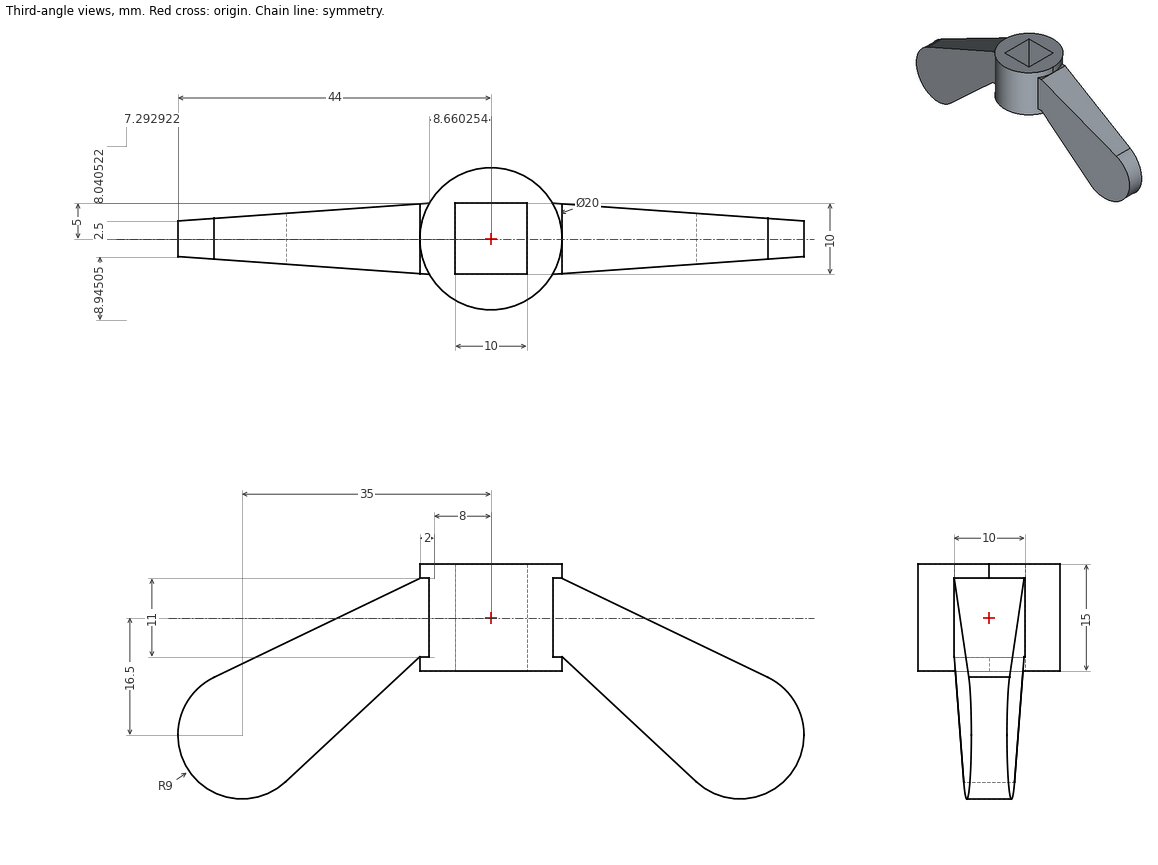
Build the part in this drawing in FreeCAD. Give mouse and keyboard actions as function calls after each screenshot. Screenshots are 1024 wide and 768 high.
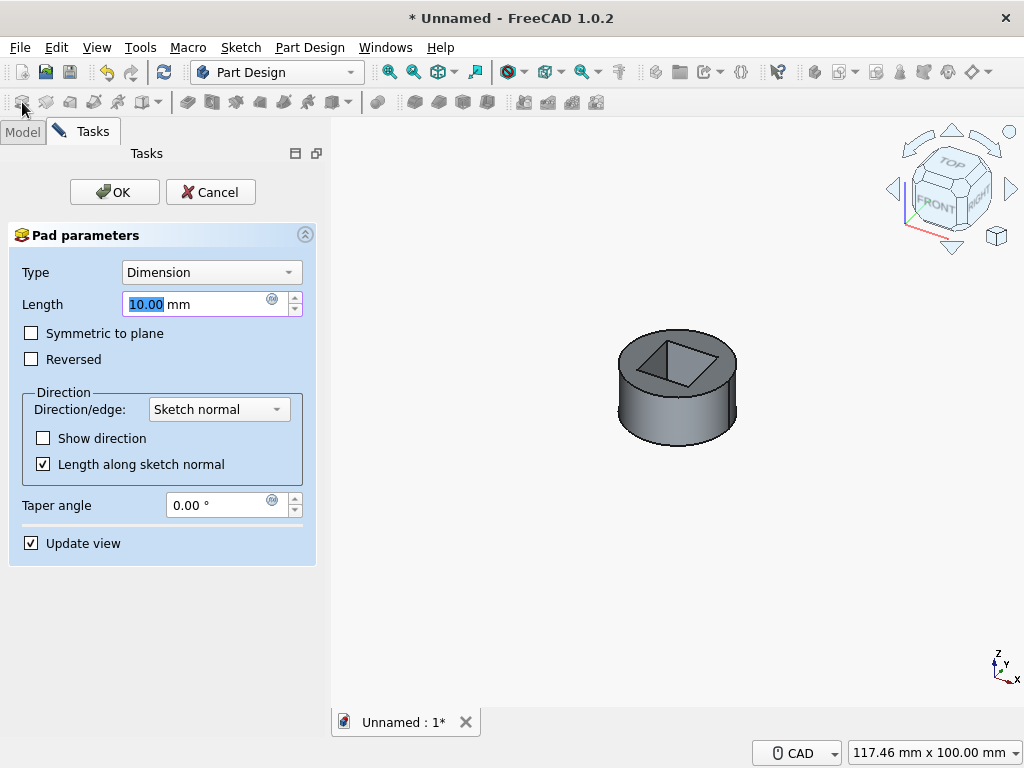
text(15)
key(Tab)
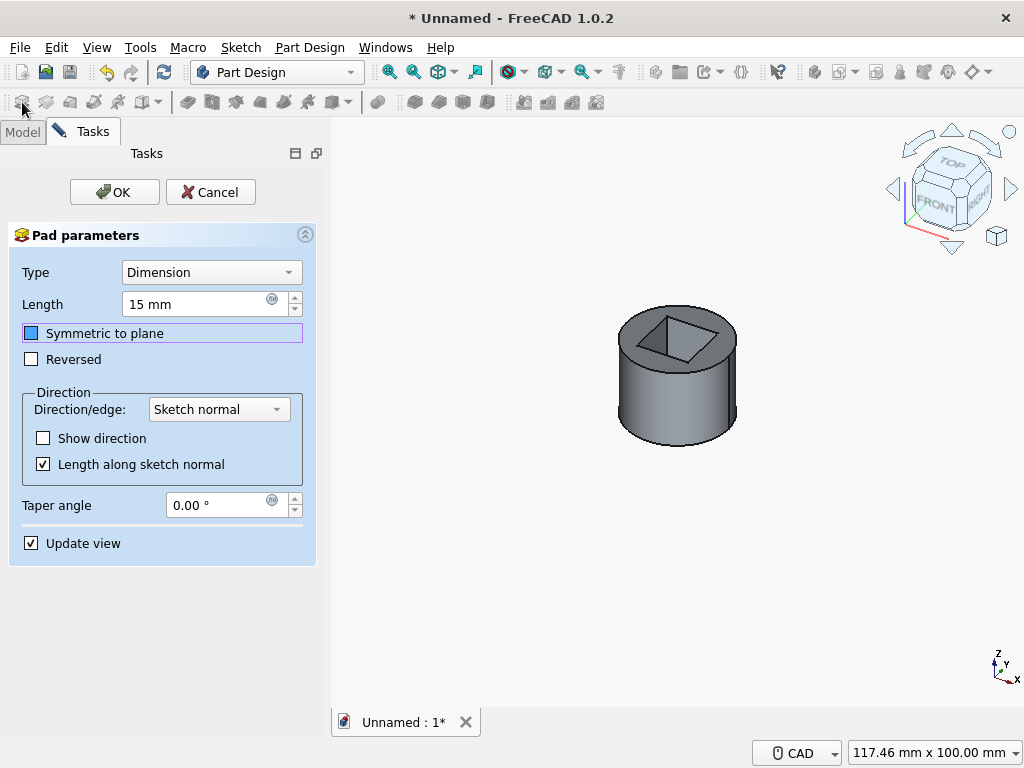
click(30, 333)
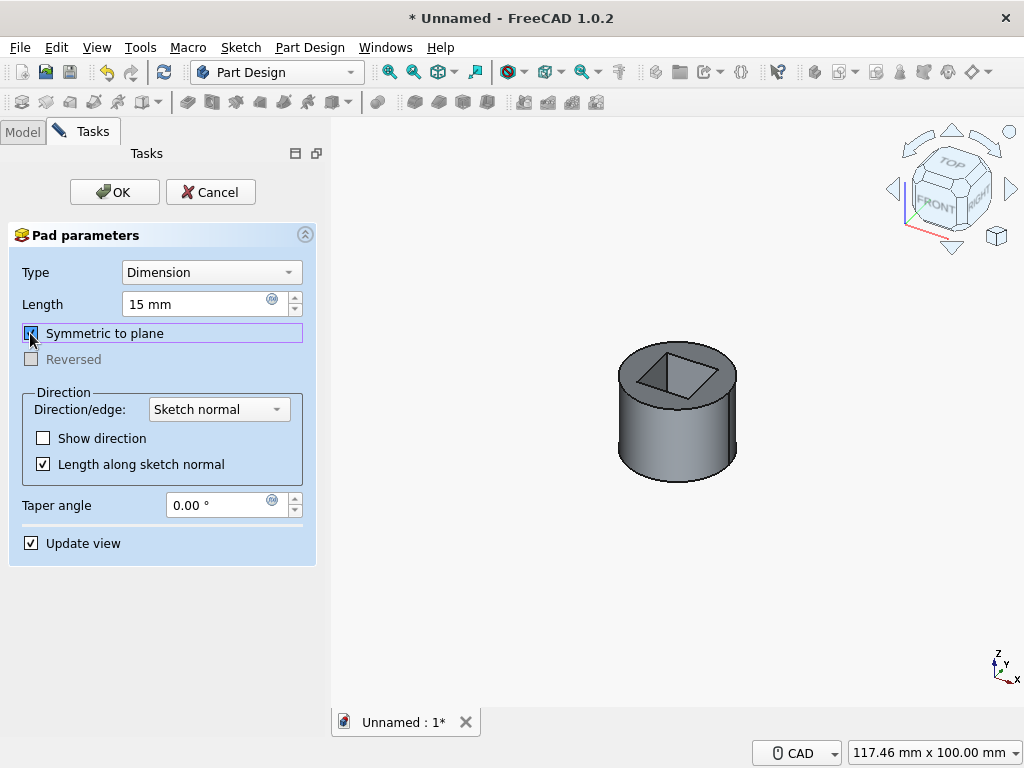
click(115, 192)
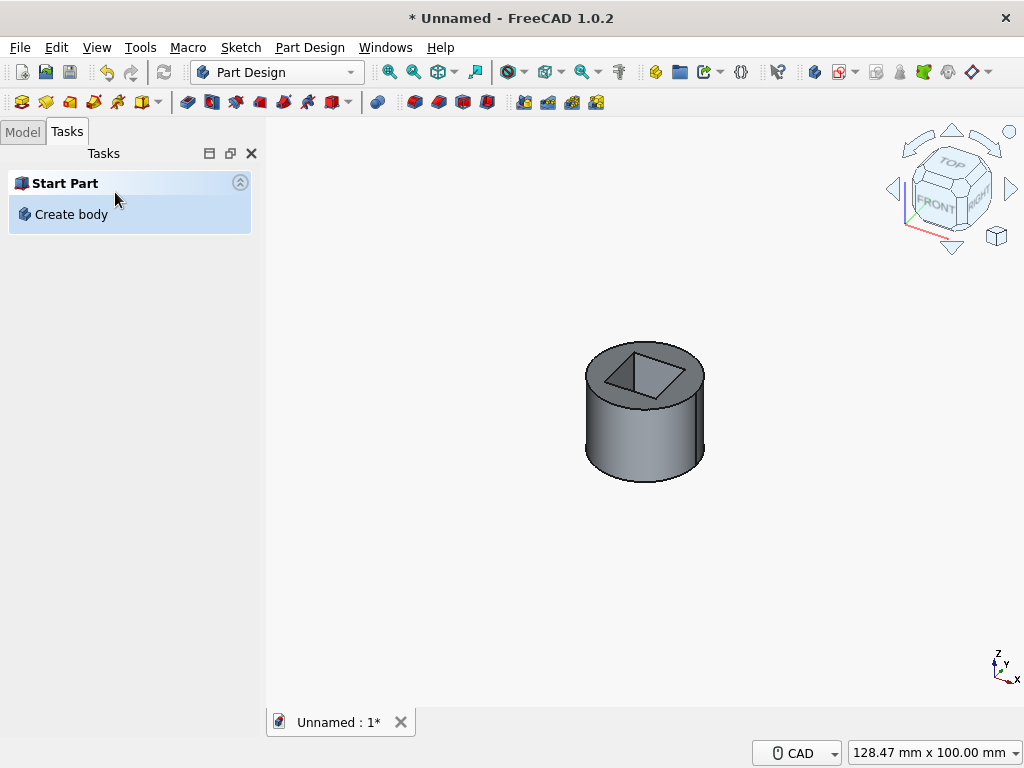
click(390, 72)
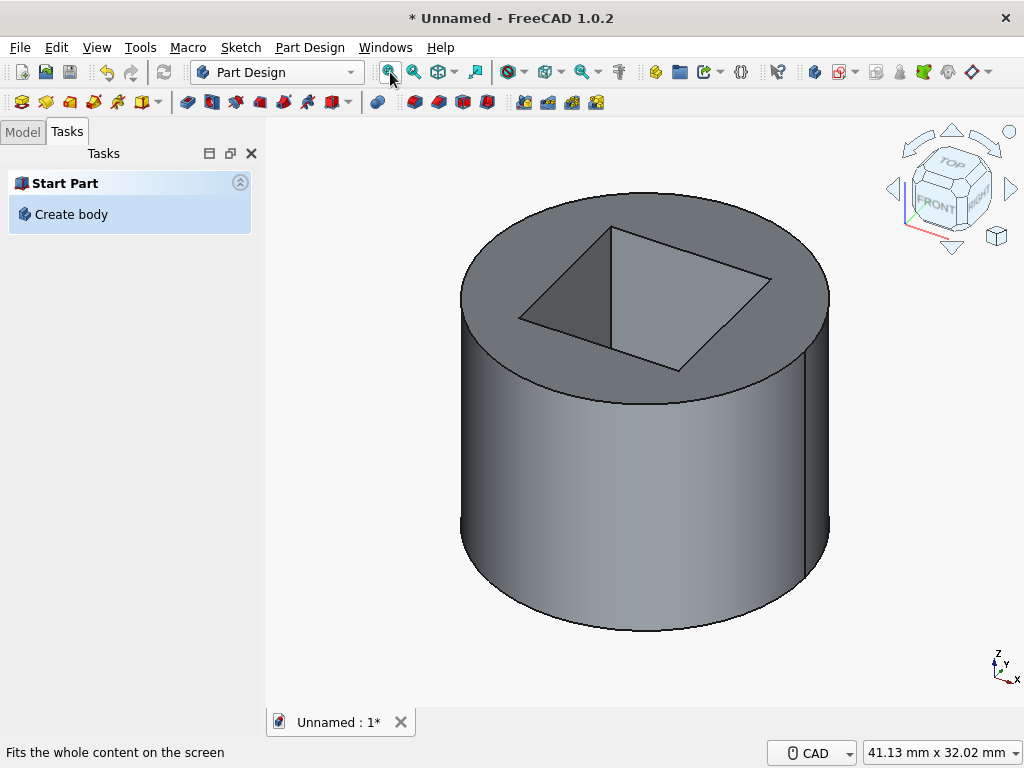
click(840, 72)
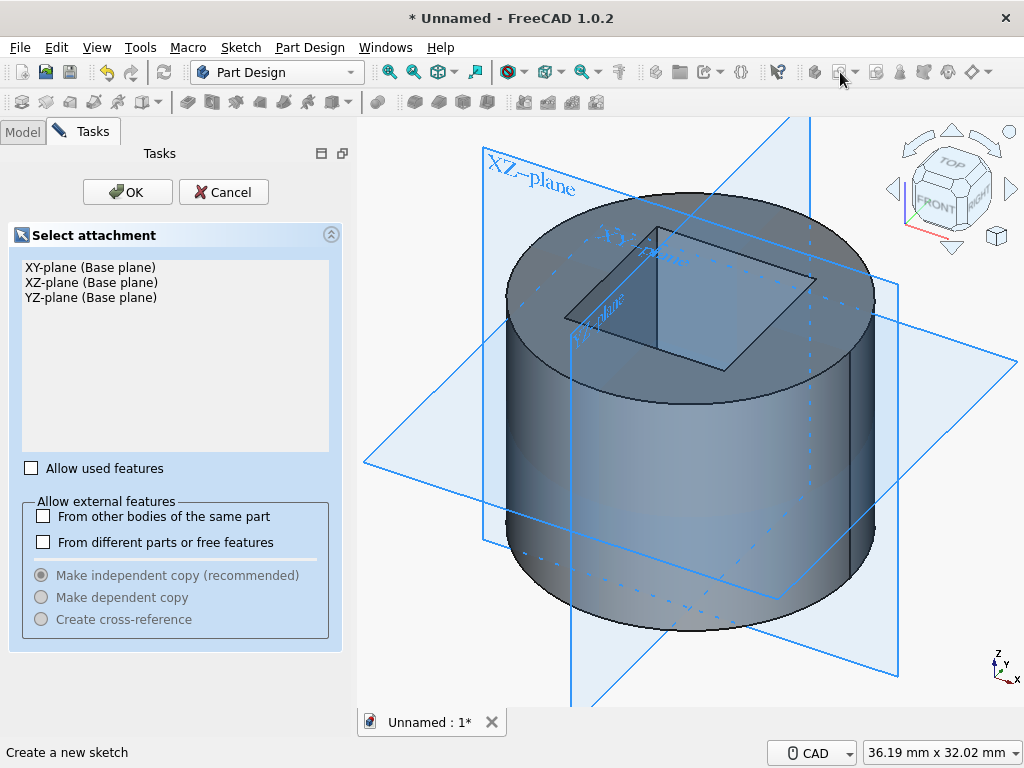
click(82, 282)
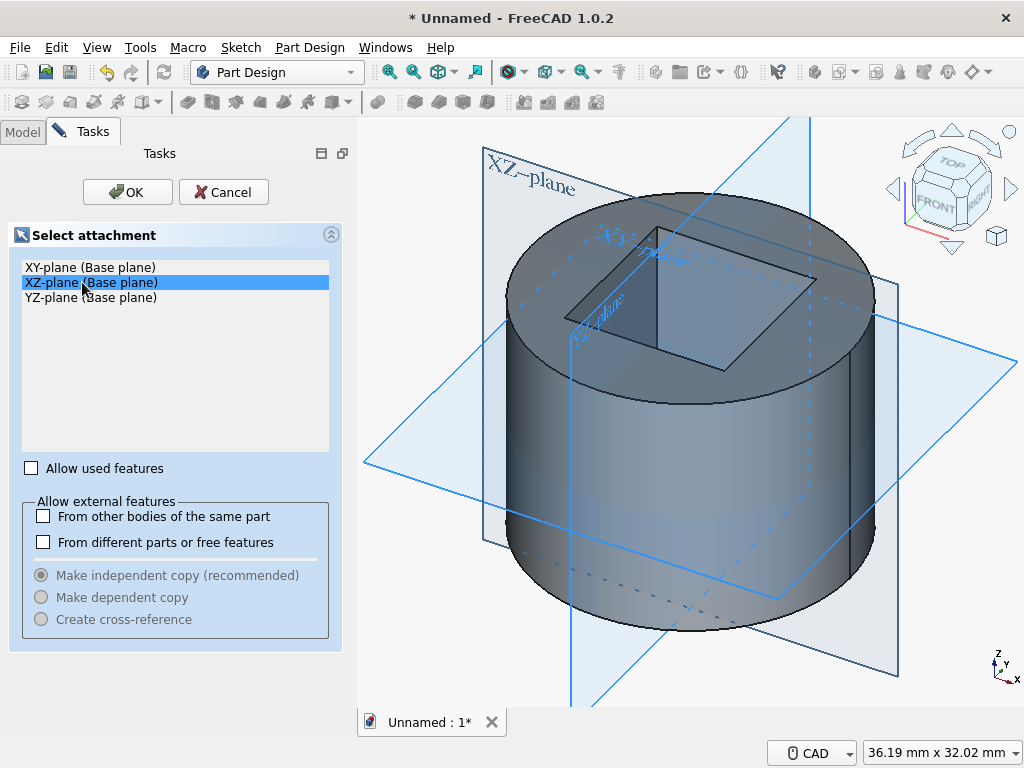
click(128, 192)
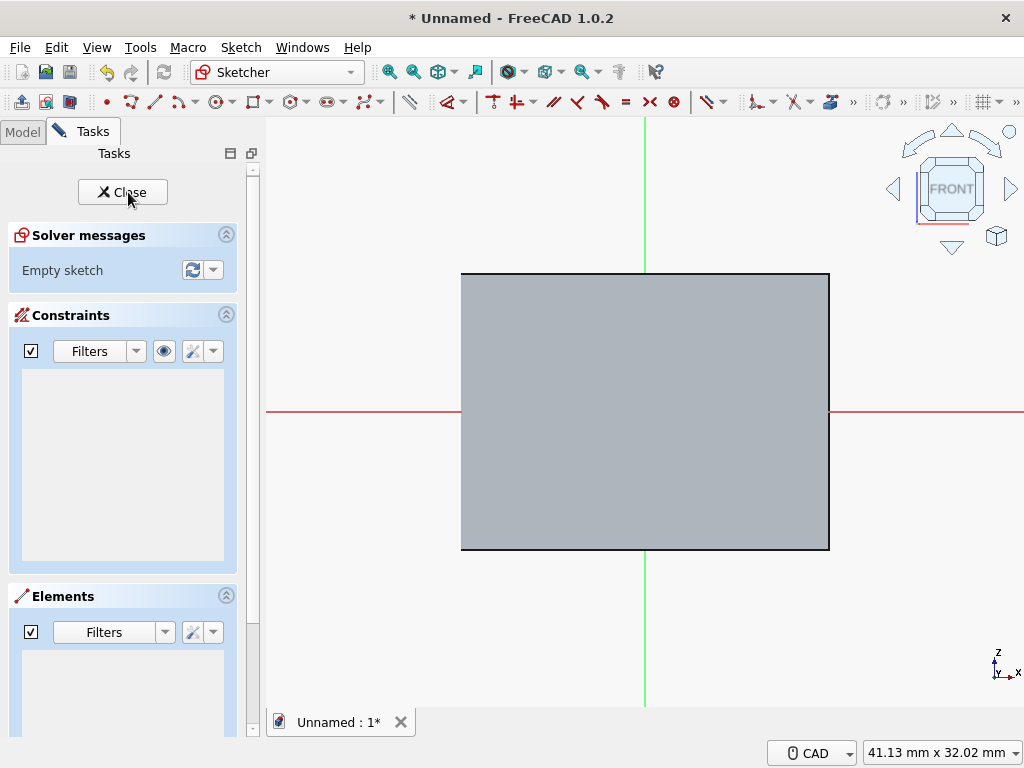
click(70, 102)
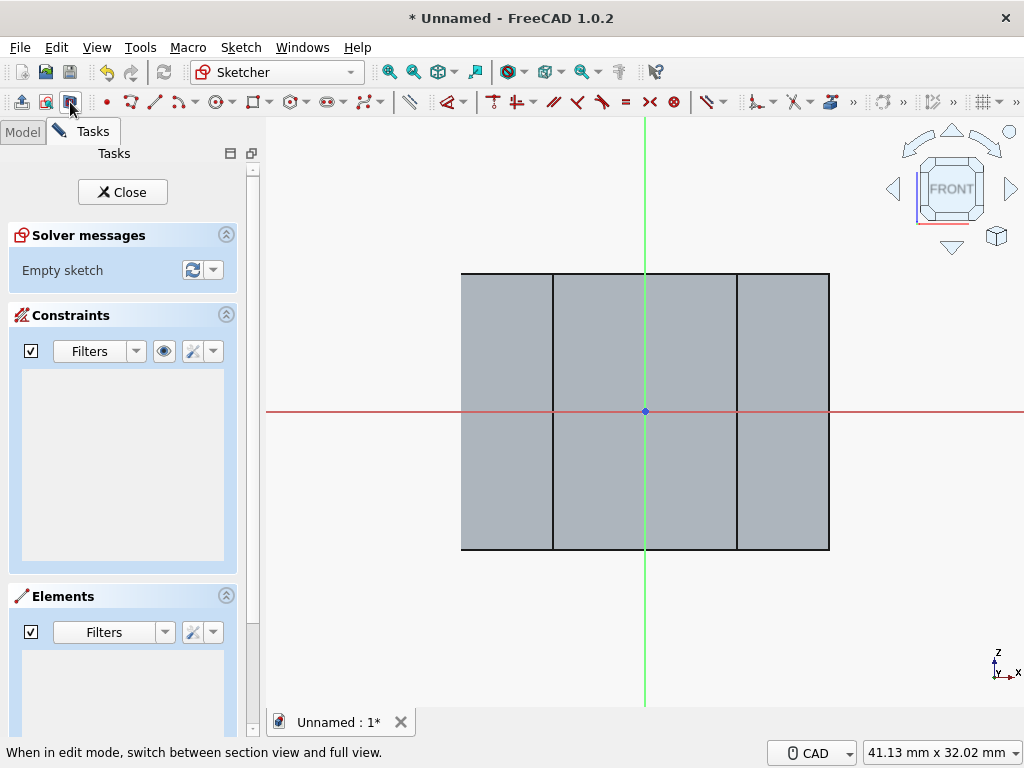
scroll(840, 280, down, 4)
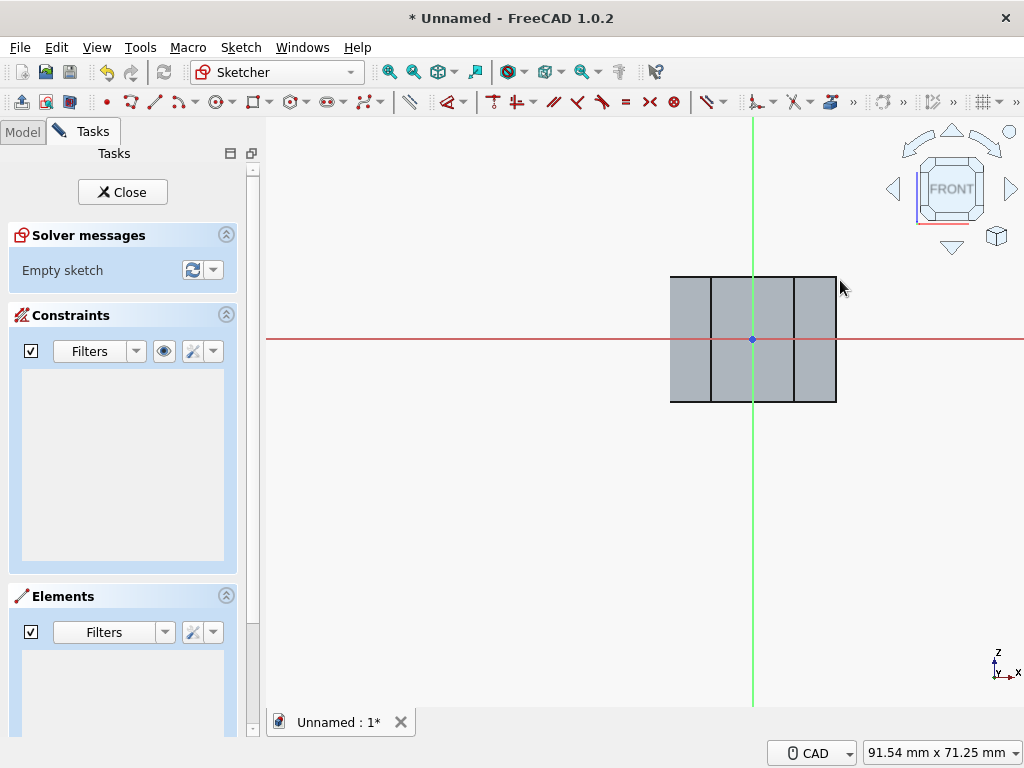
click(132, 102)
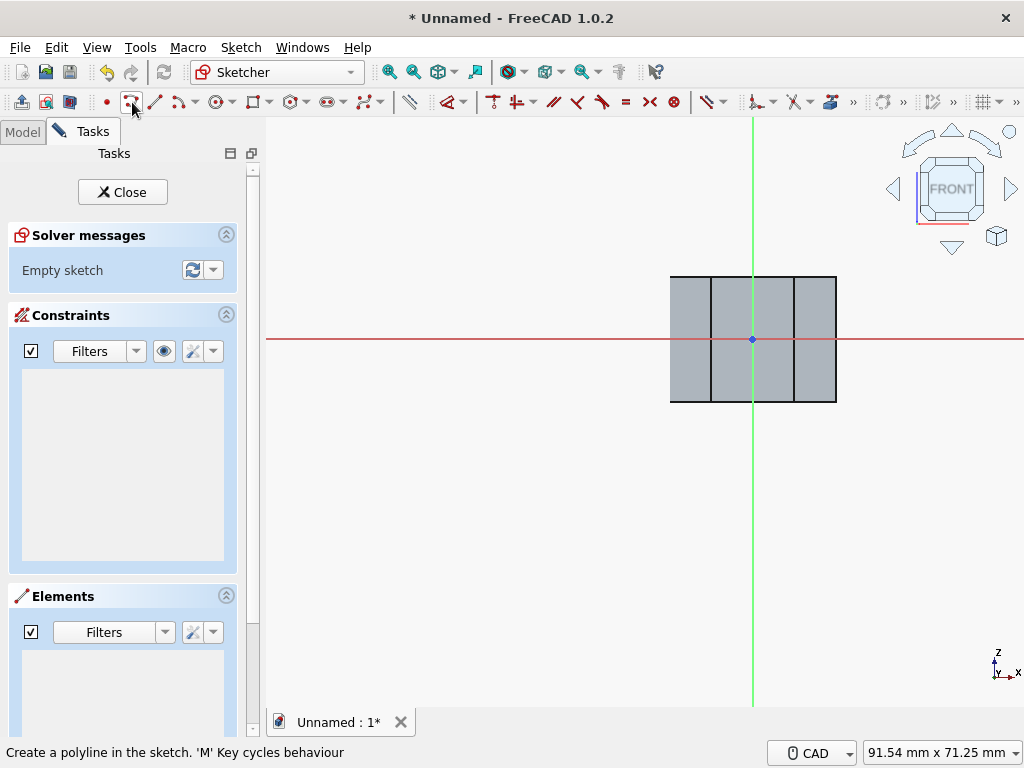
click(431, 409)
click(670, 294)
click(687, 294)
click(687, 385)
click(670, 385)
click(514, 531)
right_click(514, 531)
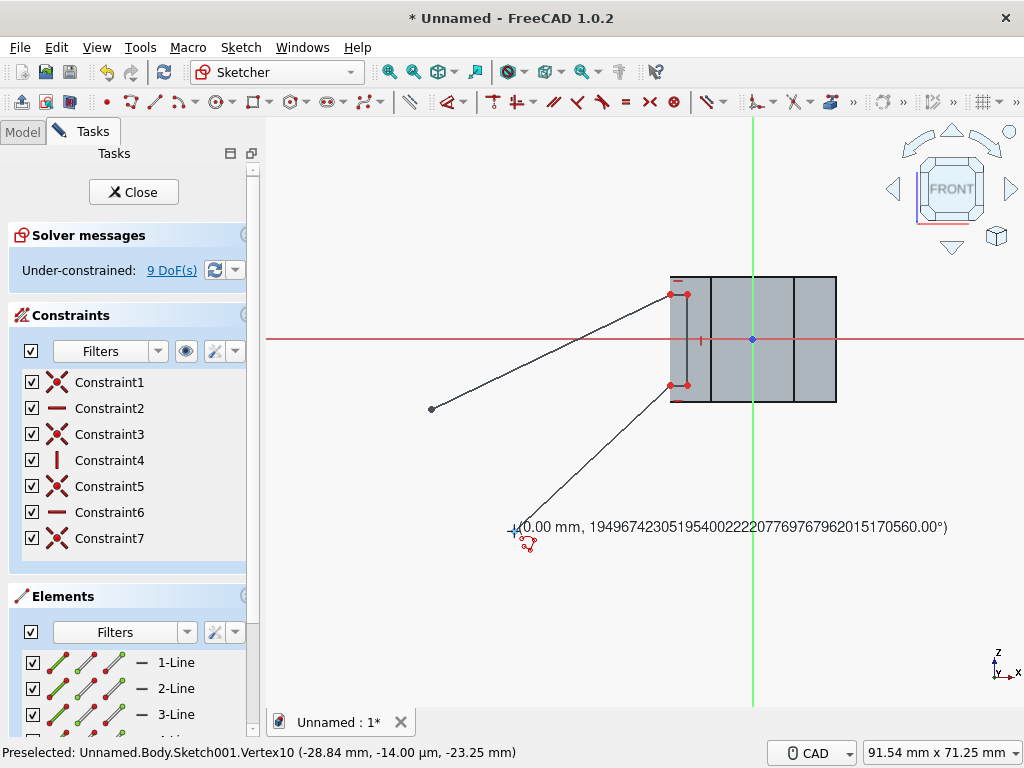
key(g)
key(3)
key(a)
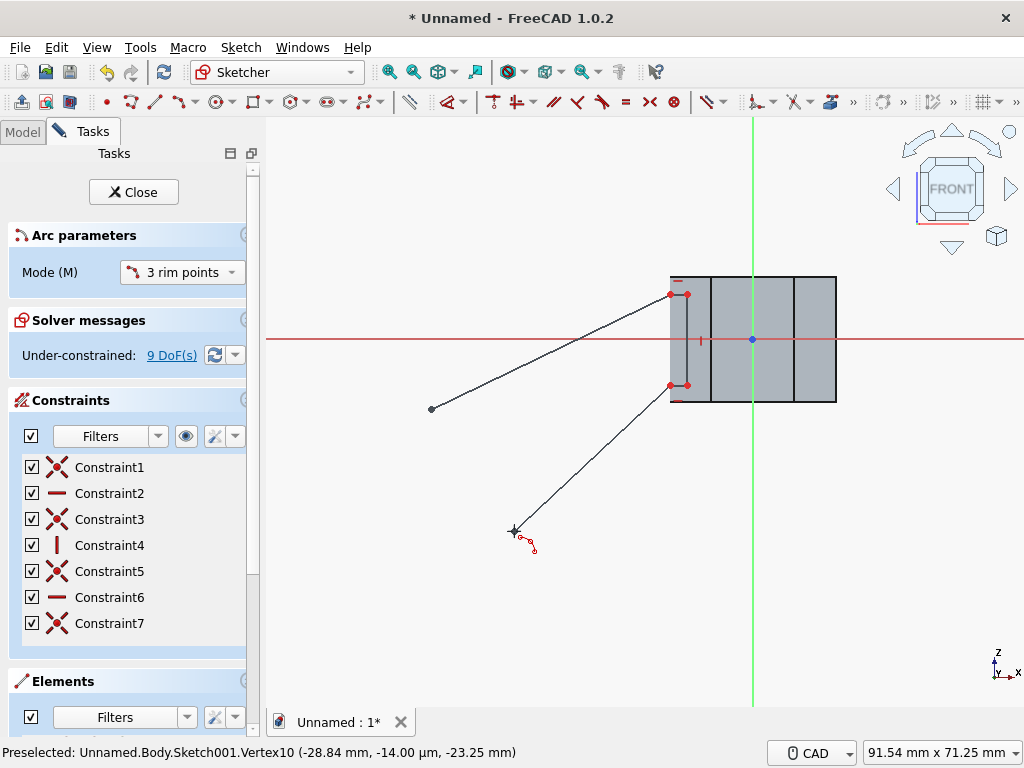
click(514, 532)
click(431, 410)
click(401, 518)
key(Escape)